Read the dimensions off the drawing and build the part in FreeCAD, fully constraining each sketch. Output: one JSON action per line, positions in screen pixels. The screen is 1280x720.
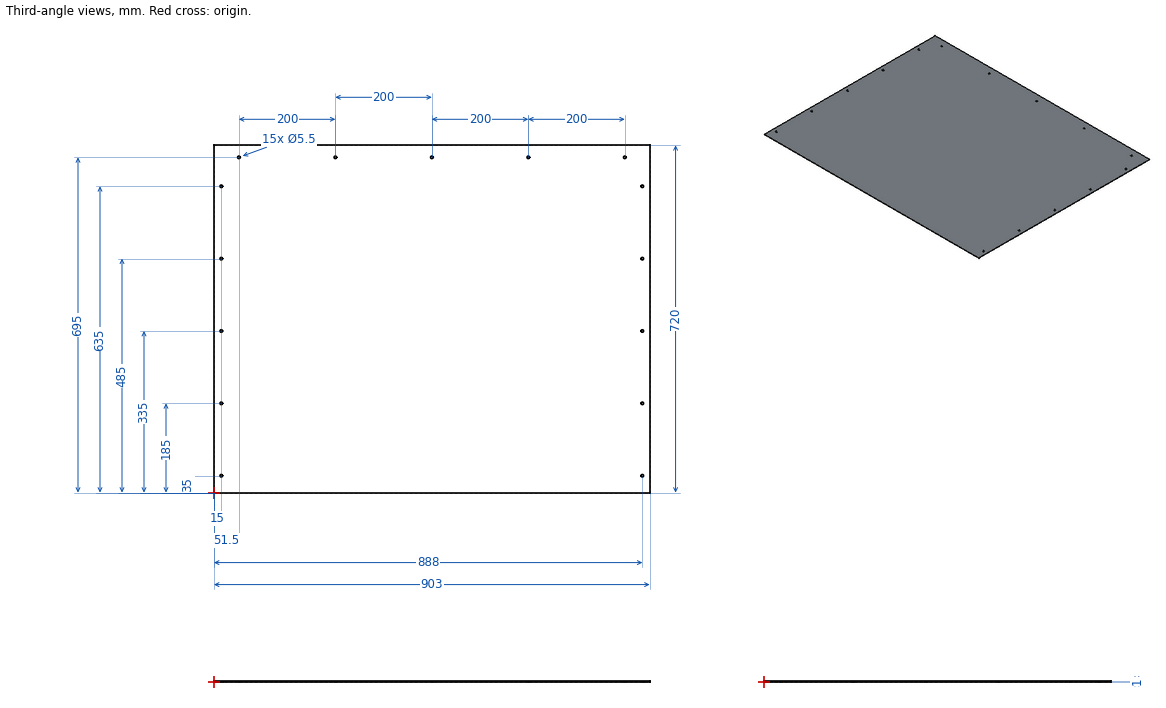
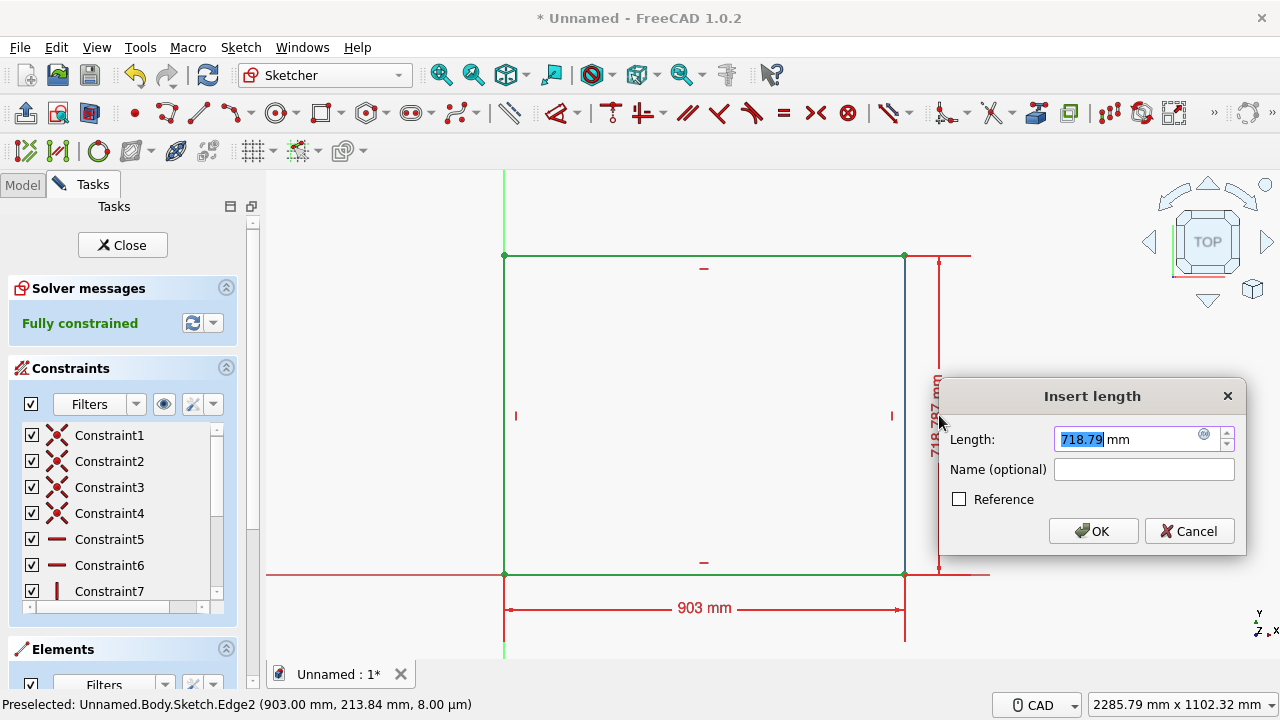
{"action": "type", "text": "720"}
{"action": "key", "text": "Return"}
{"action": "key", "text": "Escape"}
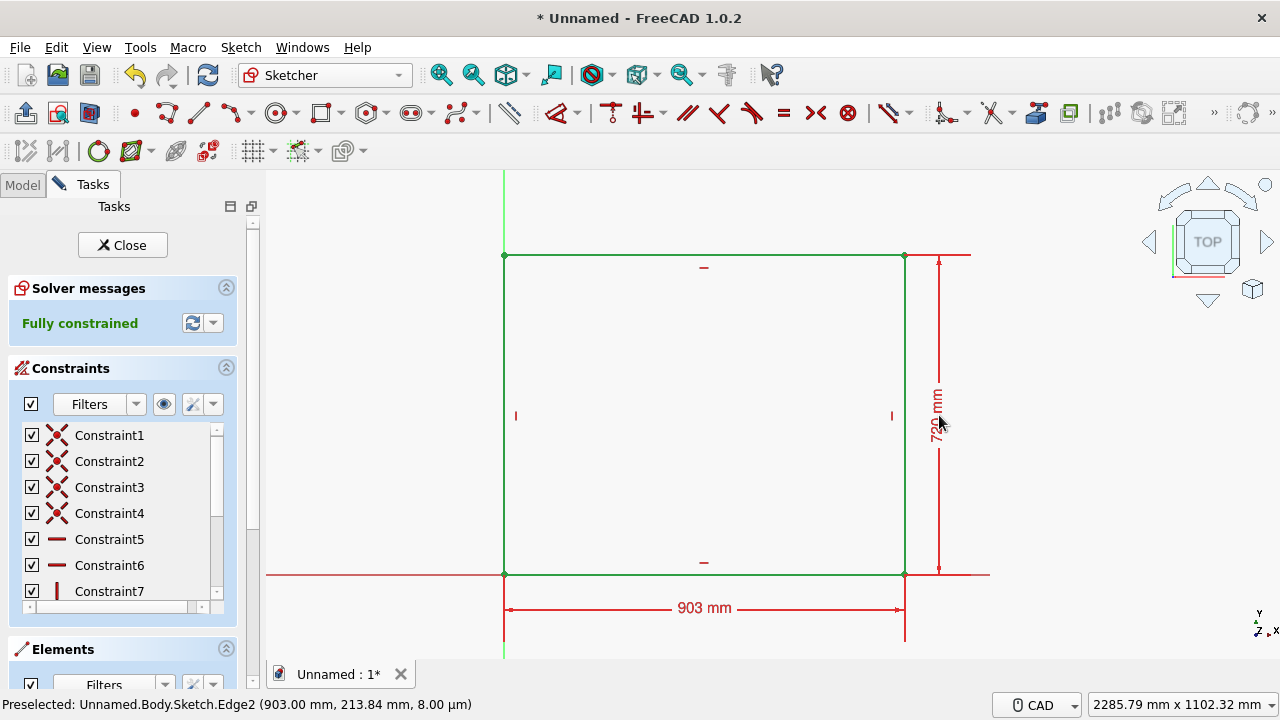
{"action": "left_click", "coordinate": [123, 245]}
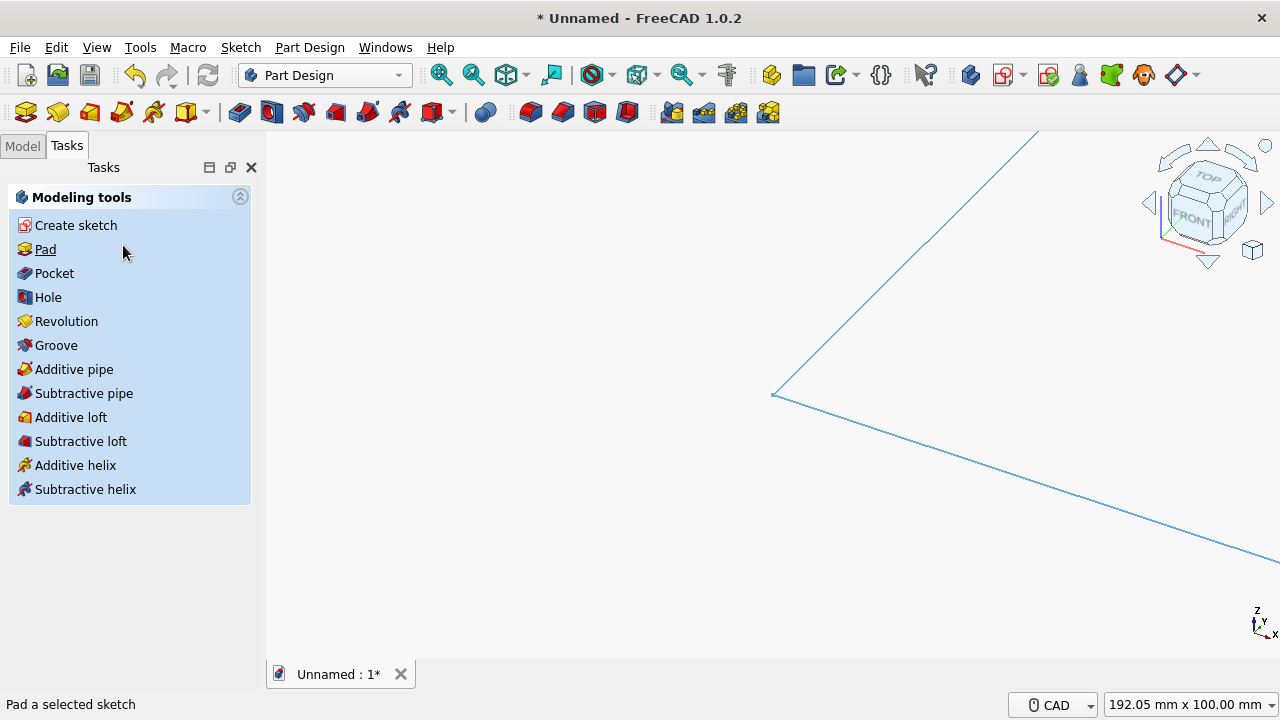
{"action": "left_click", "coordinate": [26, 112]}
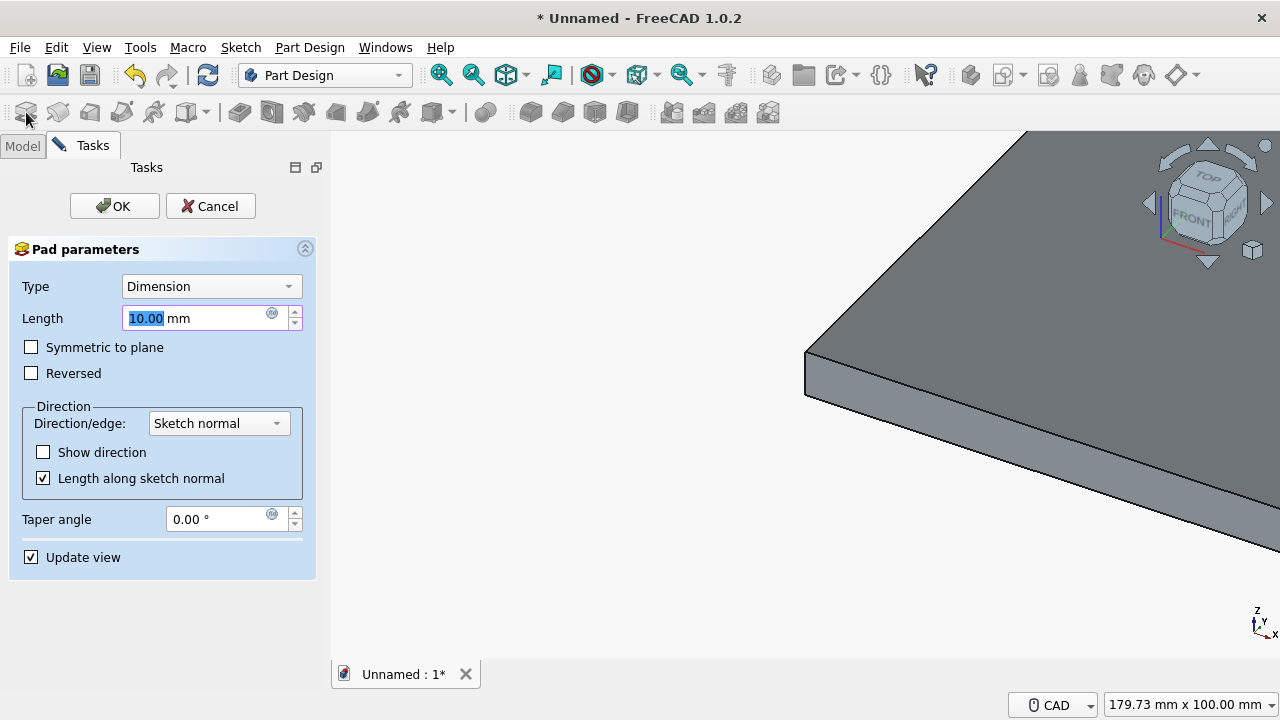
{"action": "type", "text": "1"}
{"action": "key", "text": "Tab"}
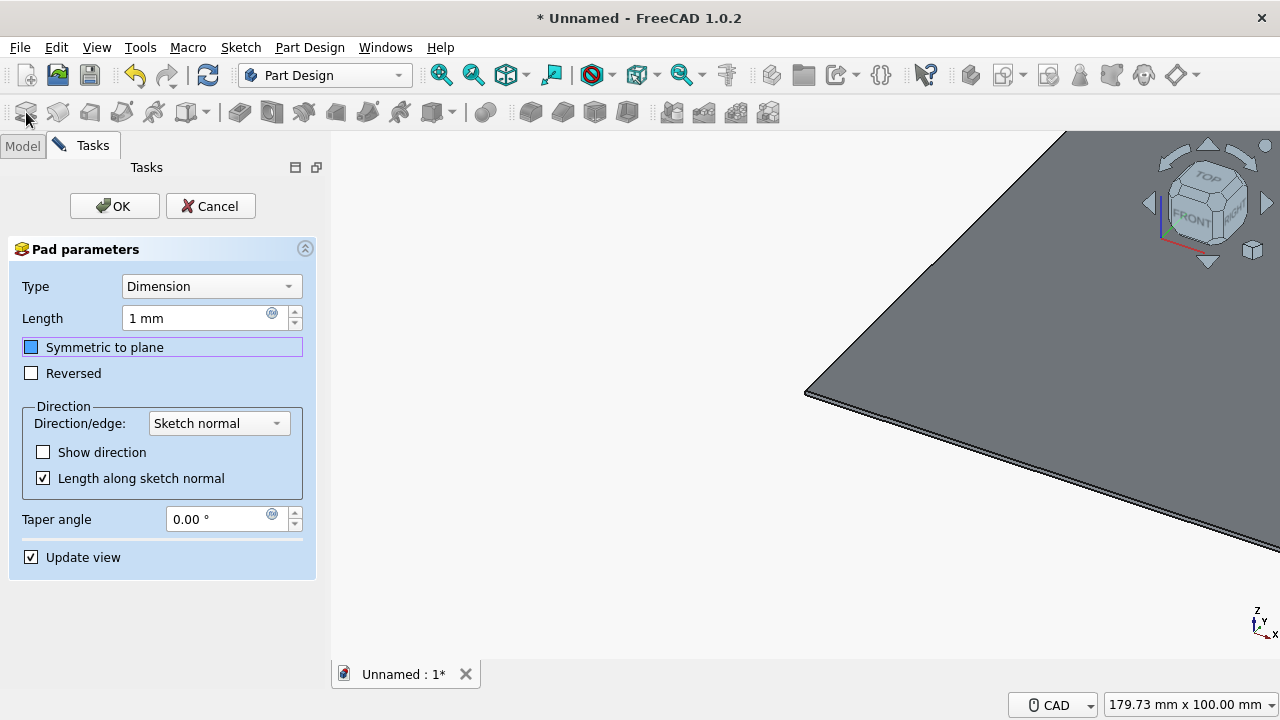
{"action": "left_click", "coordinate": [115, 206]}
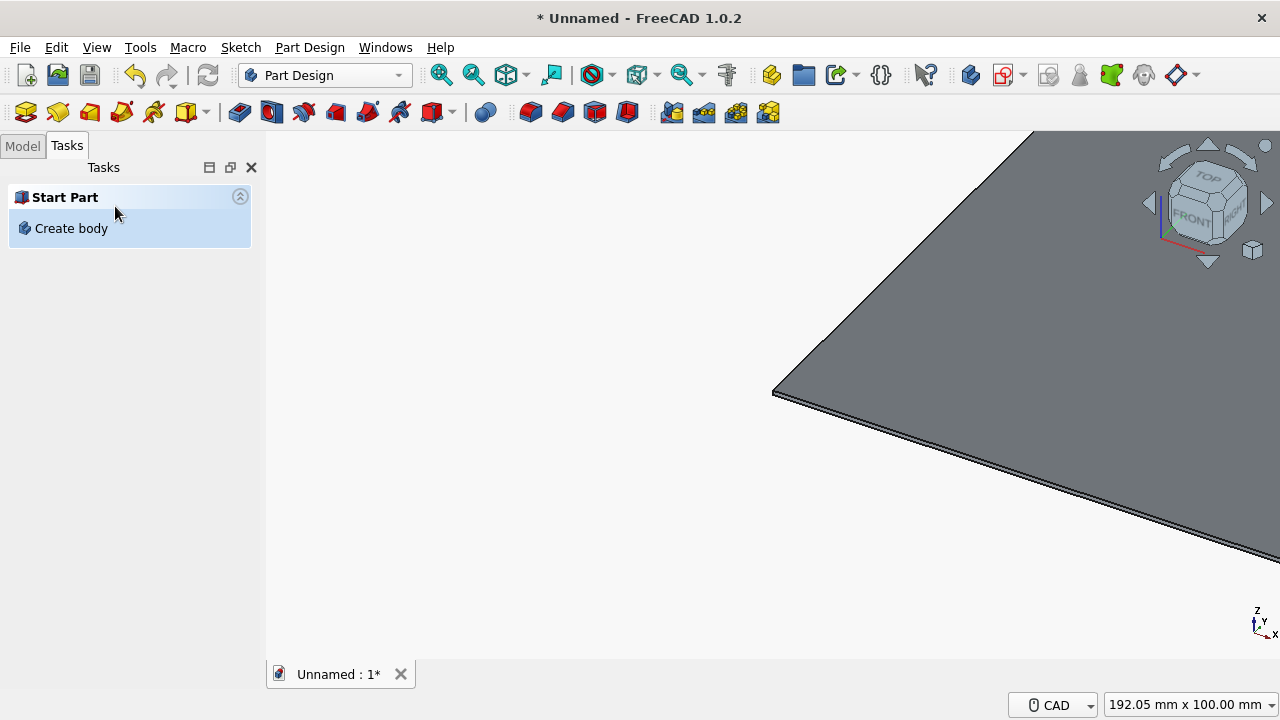
{"action": "key", "text": "v f"}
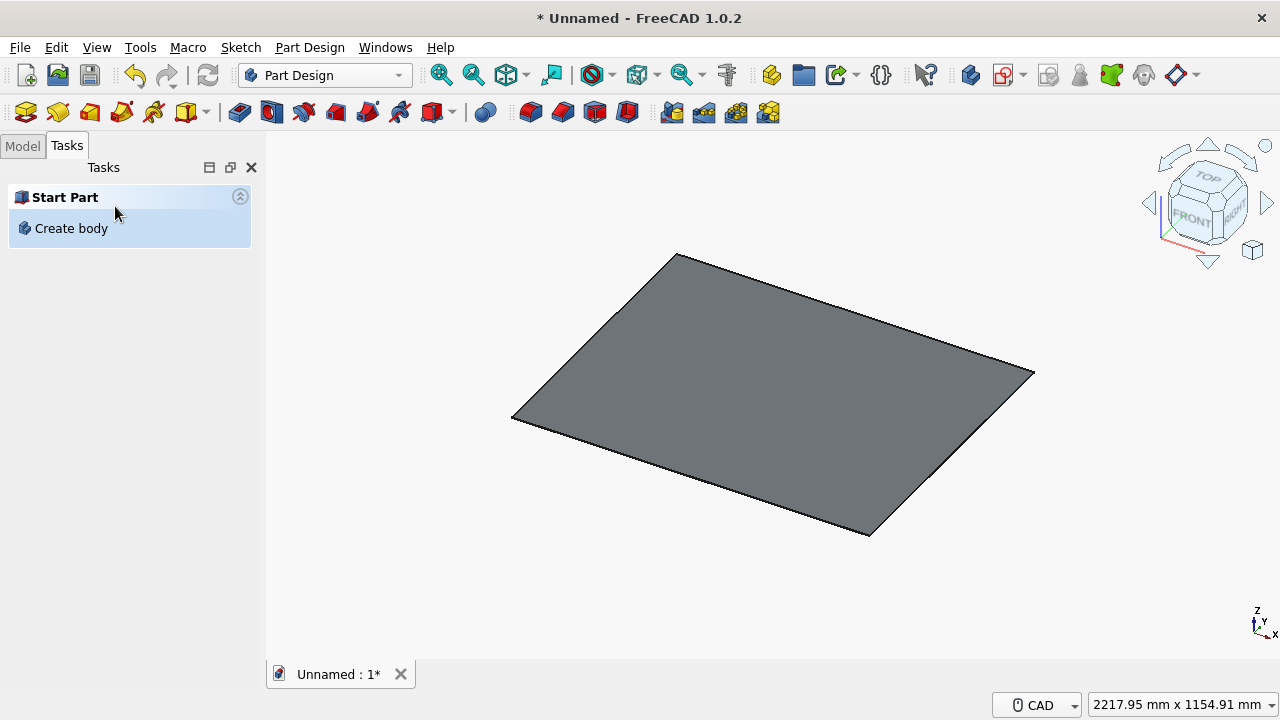
{"action": "left_click", "coordinate": [773, 394]}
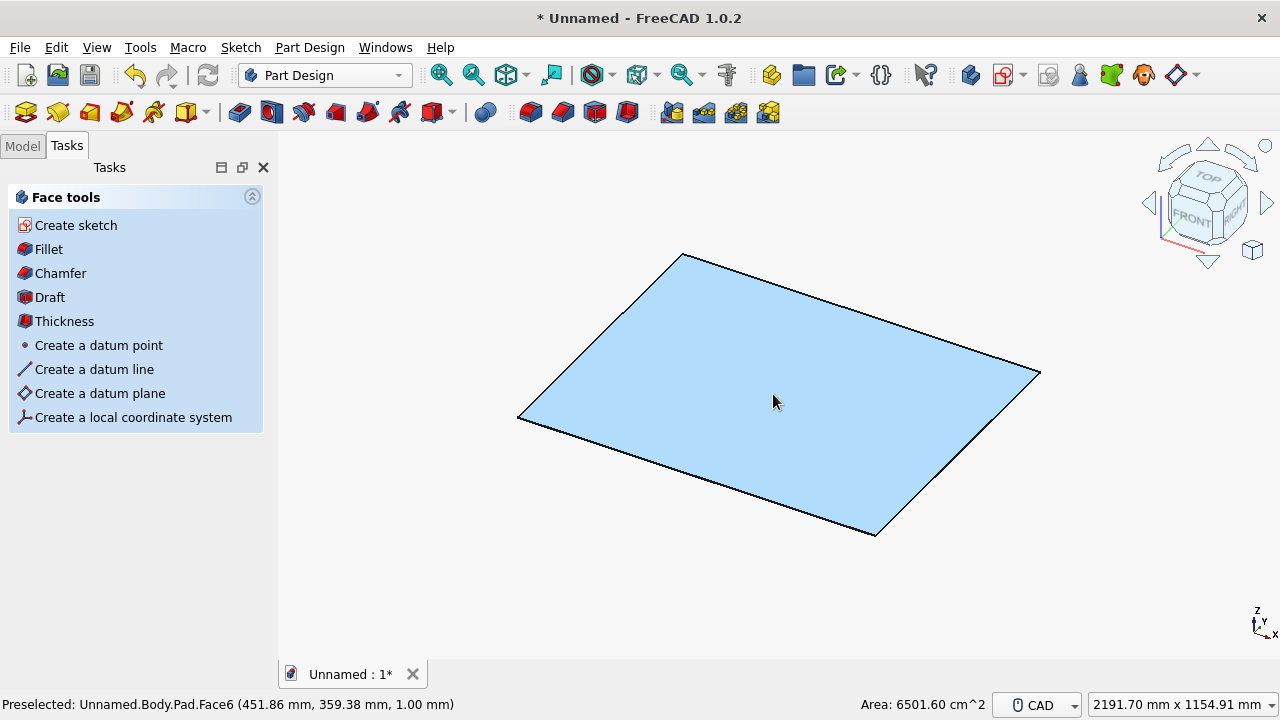
{"action": "left_click", "coordinate": [1004, 76]}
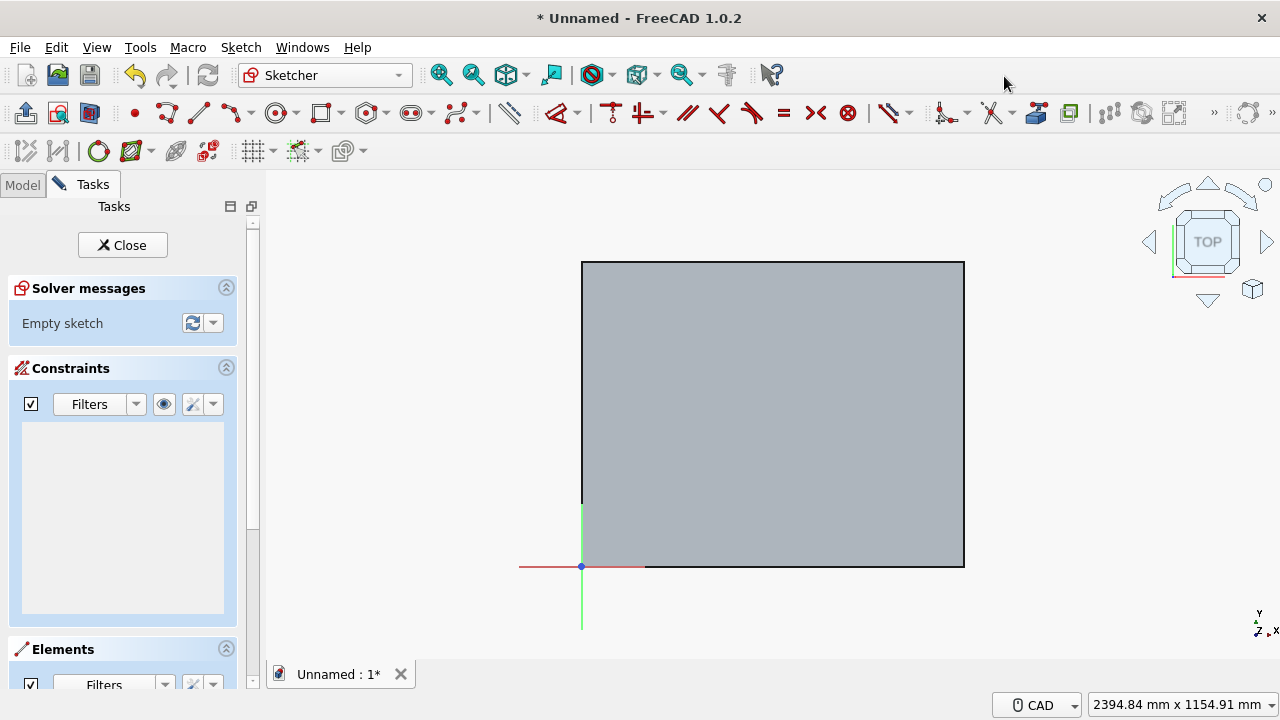
{"action": "key", "text": "g c"}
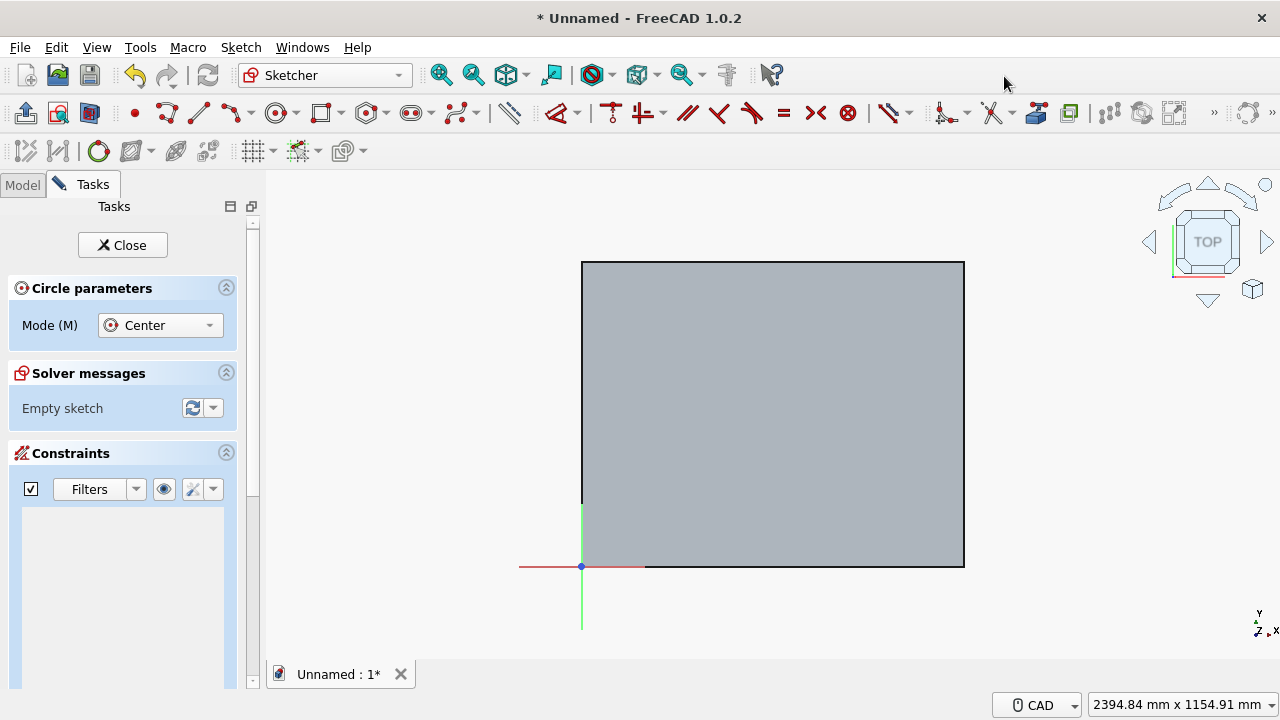
{"action": "scroll", "coordinate": [604, 273], "scroll_direction": "up", "scroll_amount": 15}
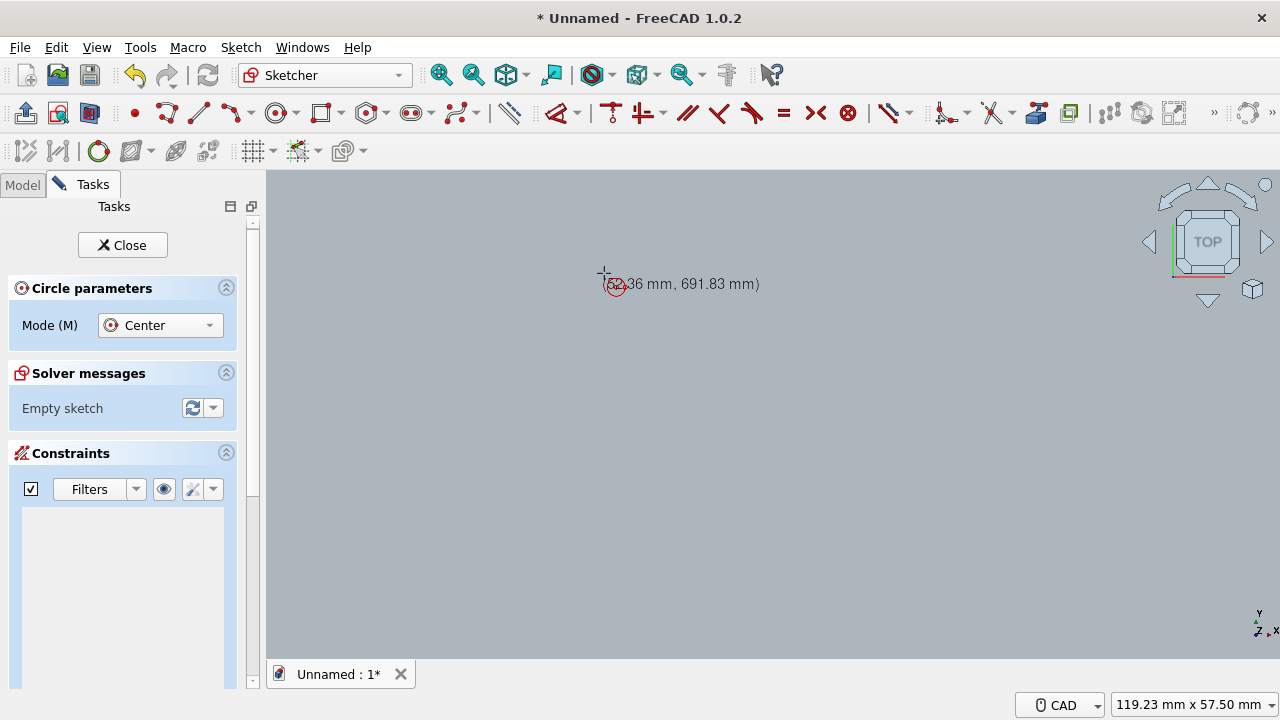
{"action": "scroll", "coordinate": [535, 268], "scroll_direction": "down", "scroll_amount": 15}